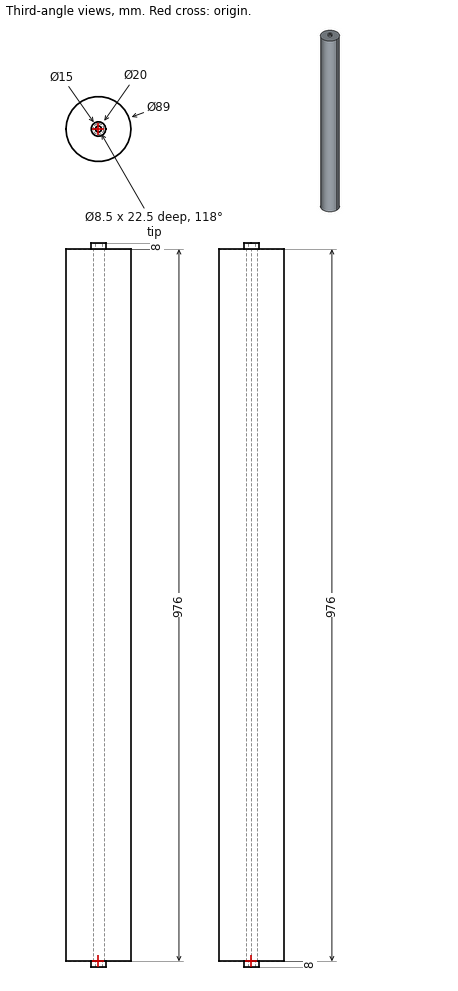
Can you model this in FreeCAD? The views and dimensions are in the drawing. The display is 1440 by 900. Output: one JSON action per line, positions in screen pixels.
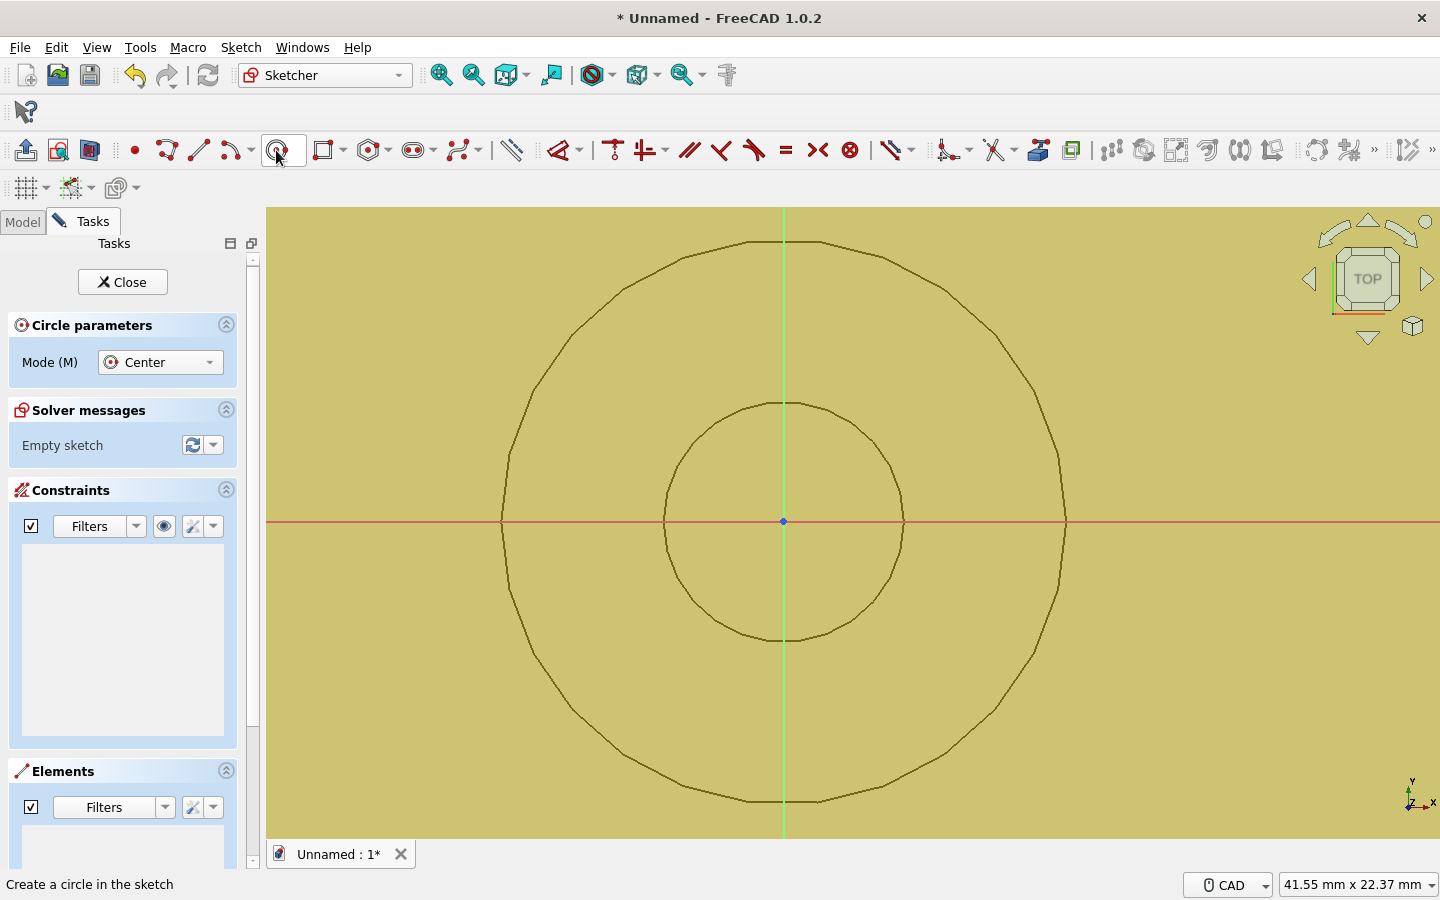
{"action": "left_click", "coordinate": [784, 522]}
{"action": "left_click", "coordinate": [934, 372]}
{"action": "key", "text": "Escape"}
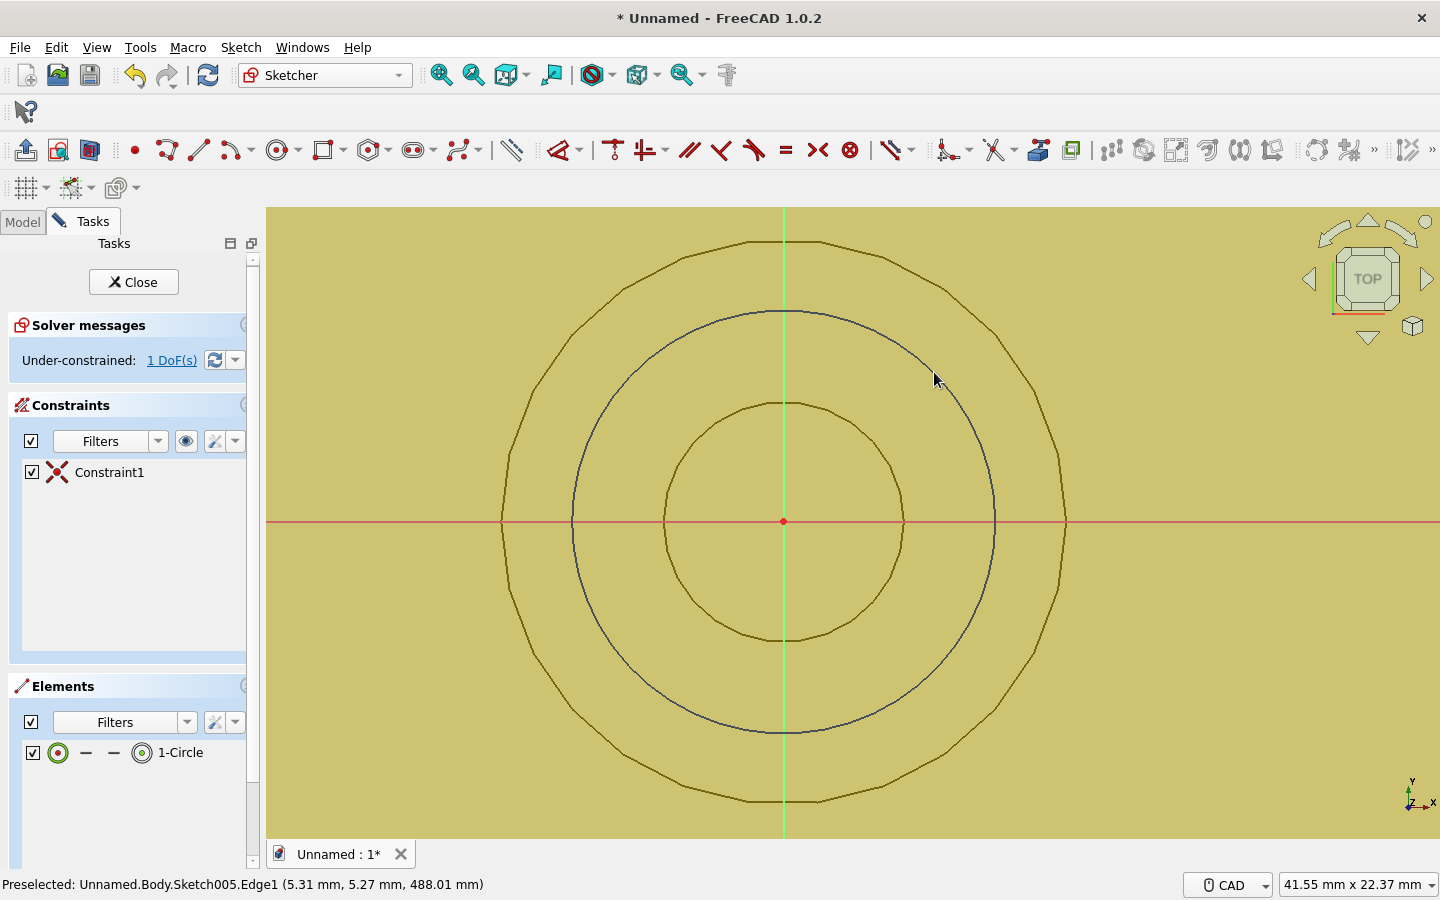
{"action": "left_click", "coordinate": [558, 150]}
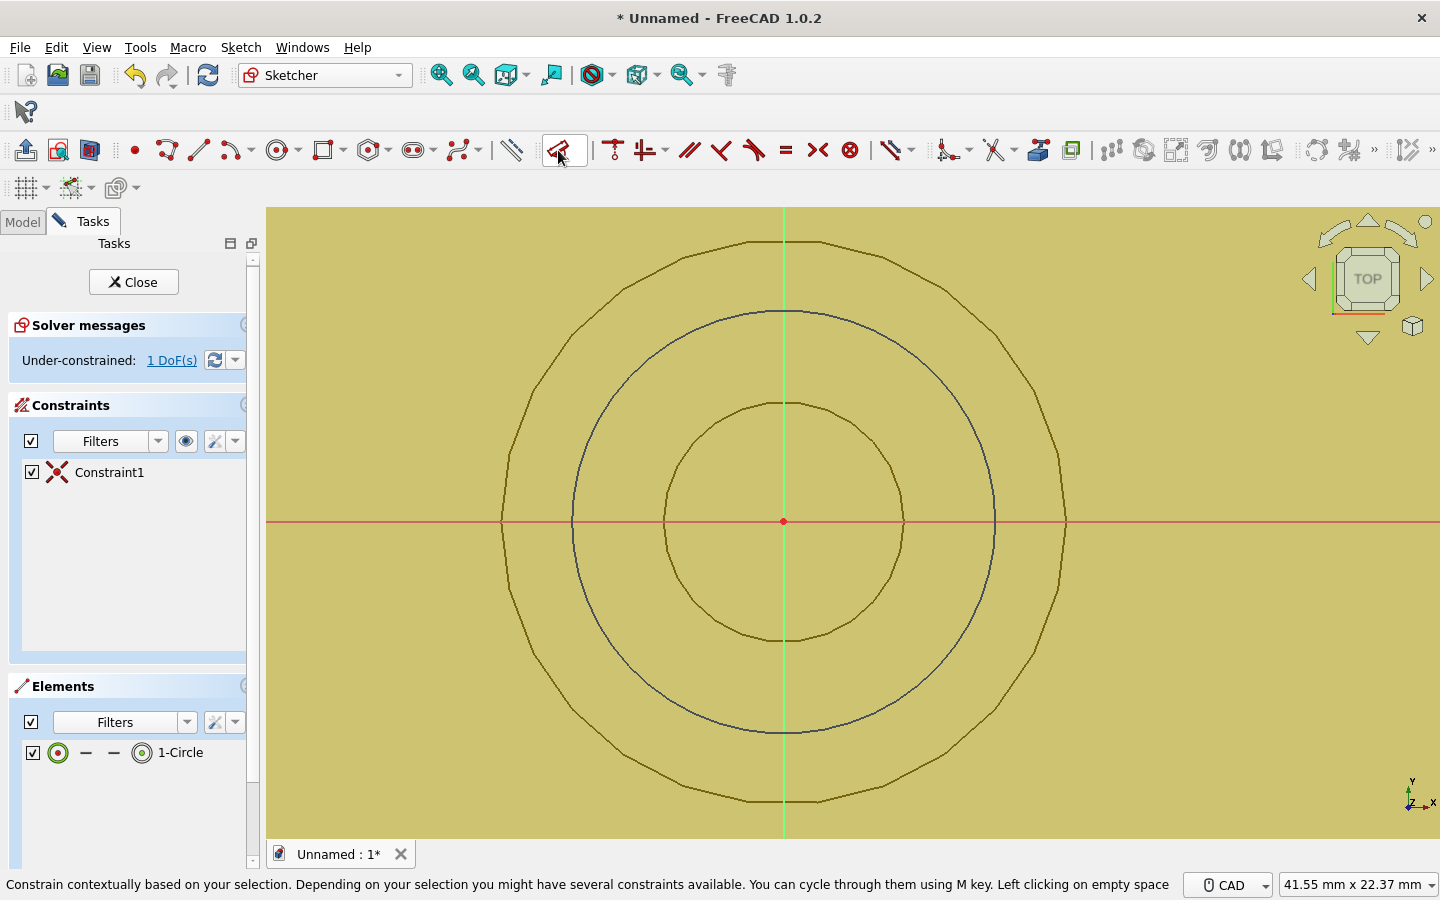
{"action": "left_click", "coordinate": [933, 372]}
{"action": "left_click", "coordinate": [956, 349]}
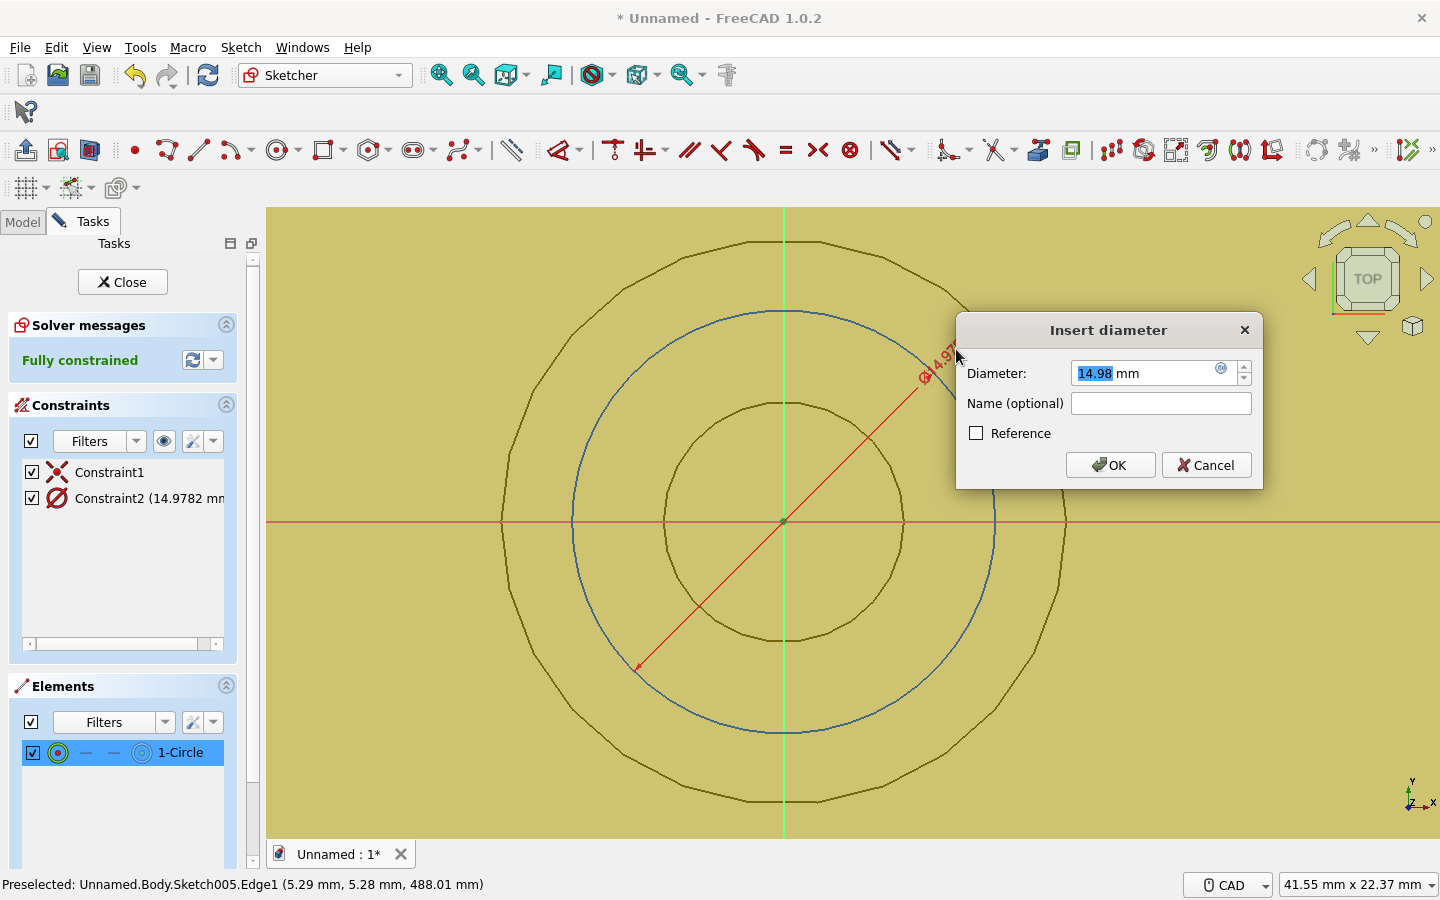
{"action": "type", "text": "15"}
{"action": "key", "text": "Return"}
{"action": "key", "text": "Escape"}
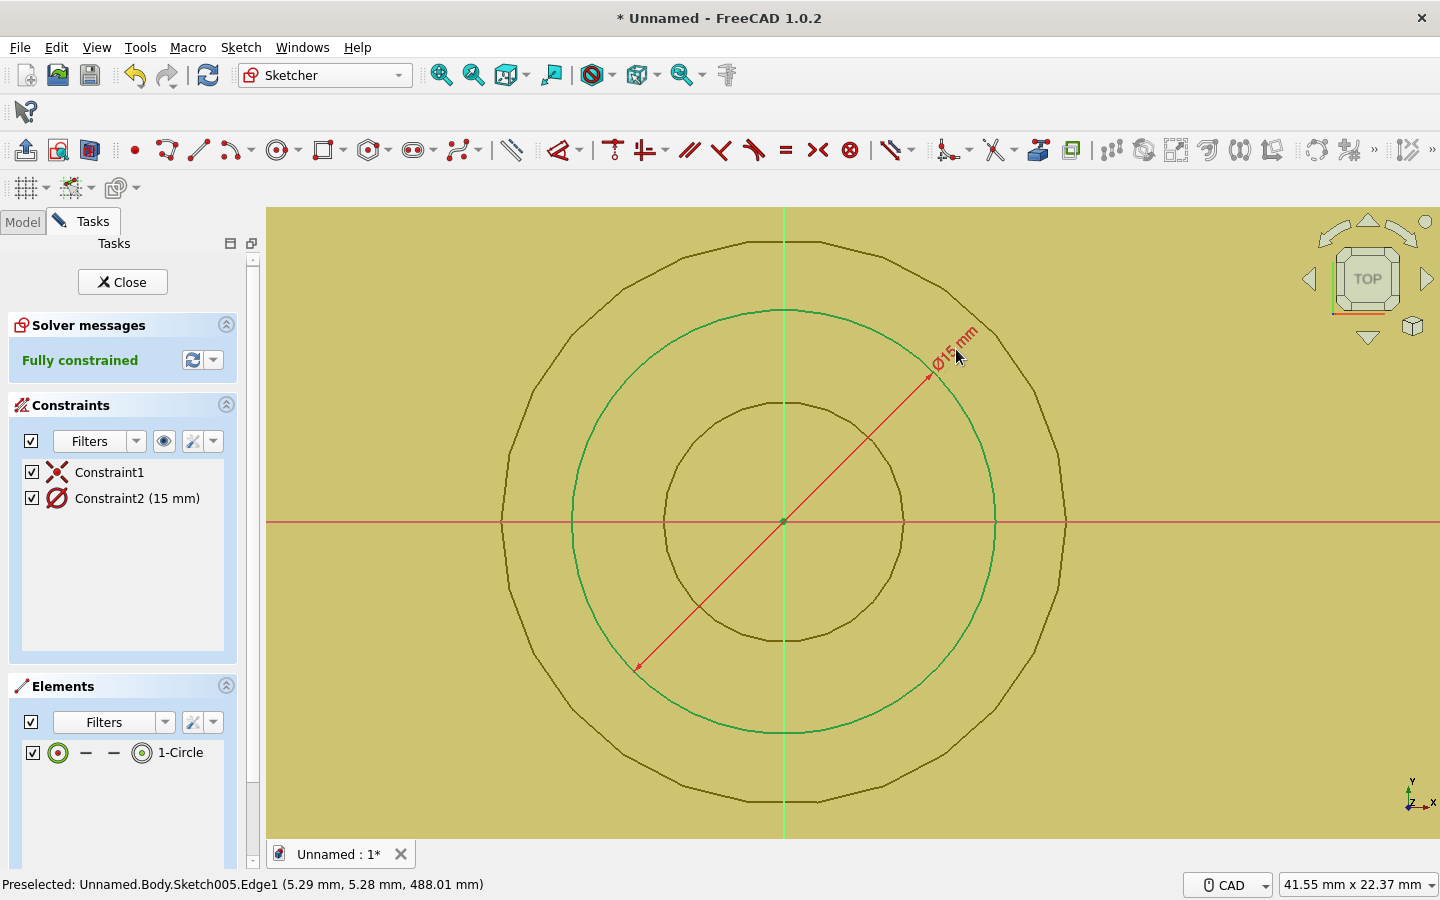
{"action": "left_click", "coordinate": [123, 282]}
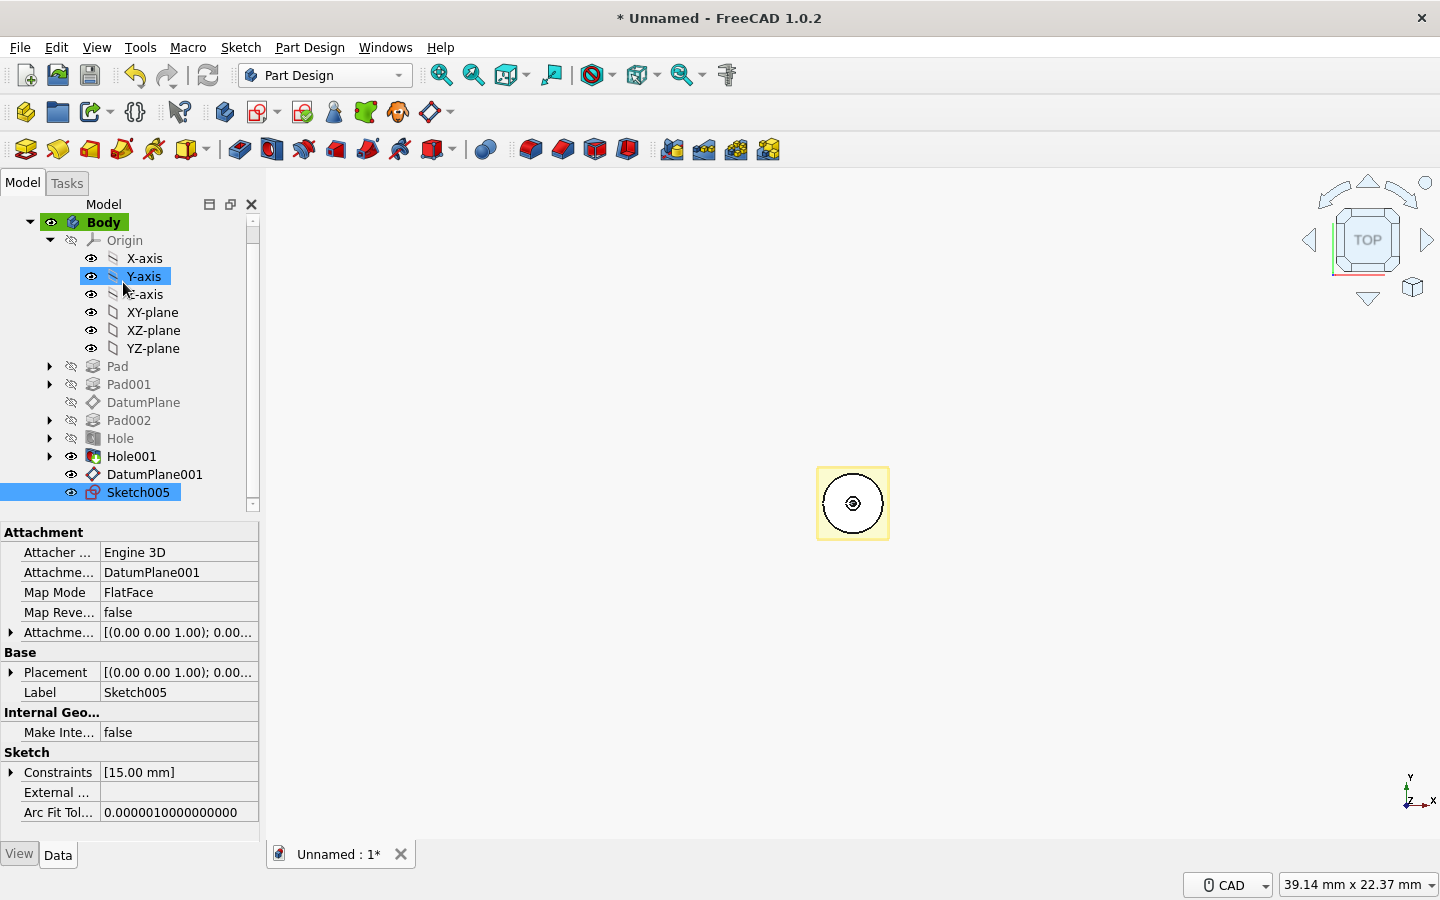
{"action": "left_click", "coordinate": [240, 150]}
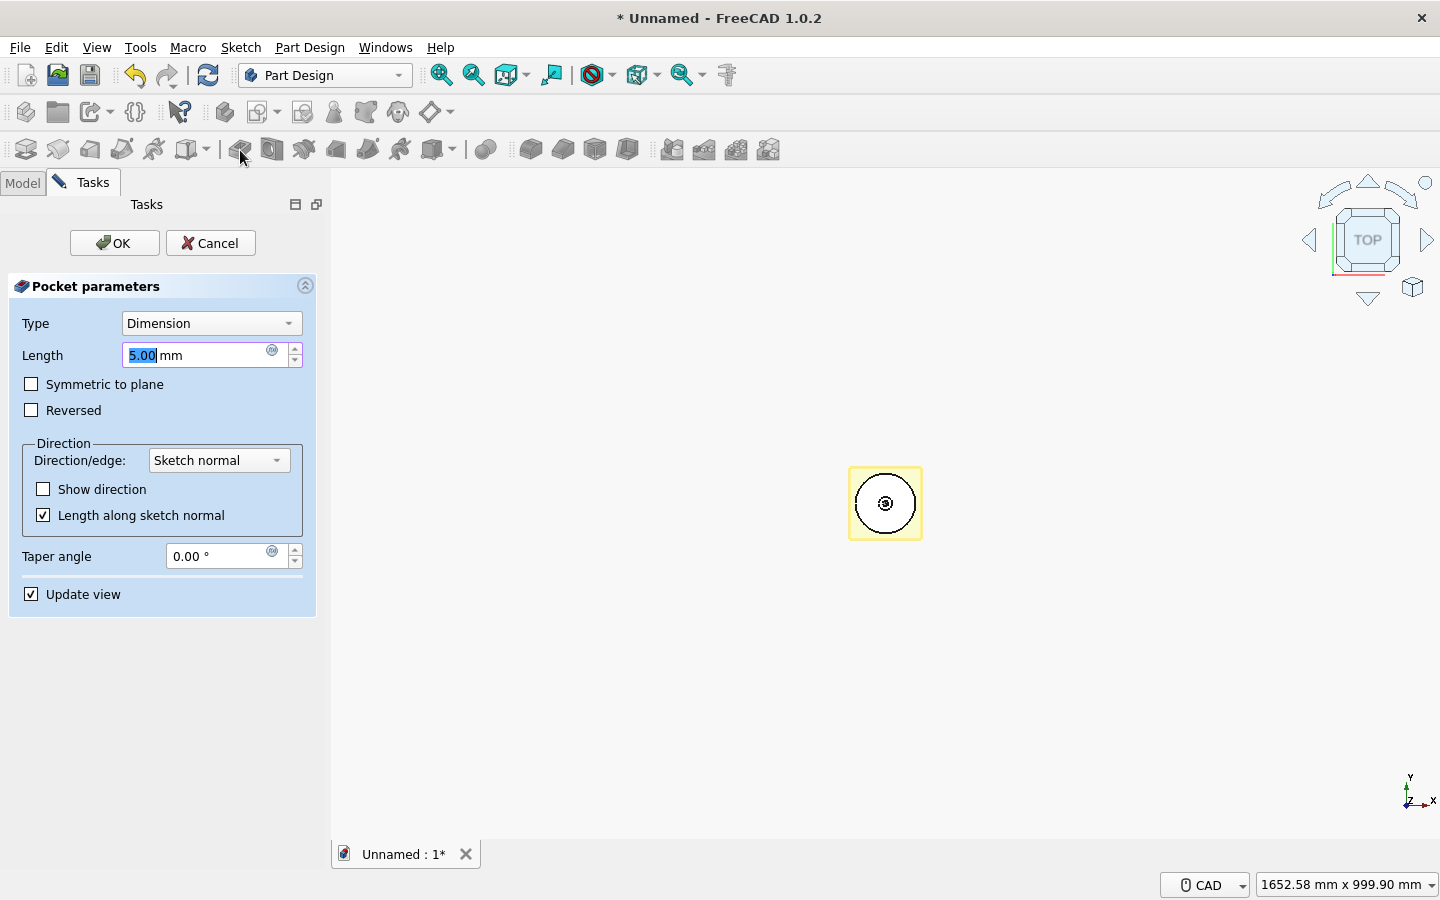
{"action": "type", "text": "976"}
{"action": "key", "text": "Tab"}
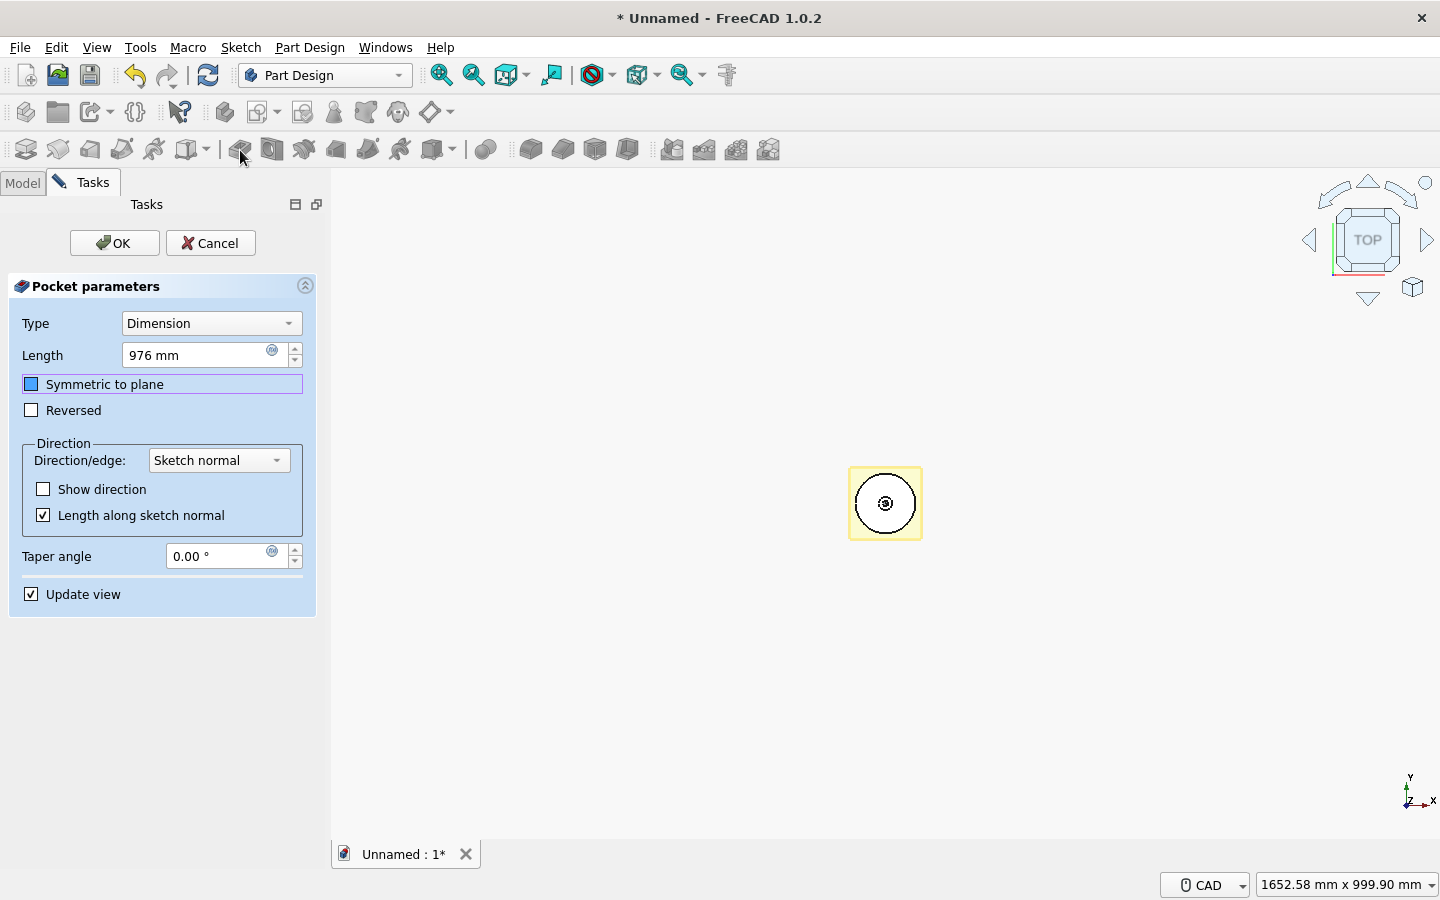
{"action": "left_click", "coordinate": [30, 384]}